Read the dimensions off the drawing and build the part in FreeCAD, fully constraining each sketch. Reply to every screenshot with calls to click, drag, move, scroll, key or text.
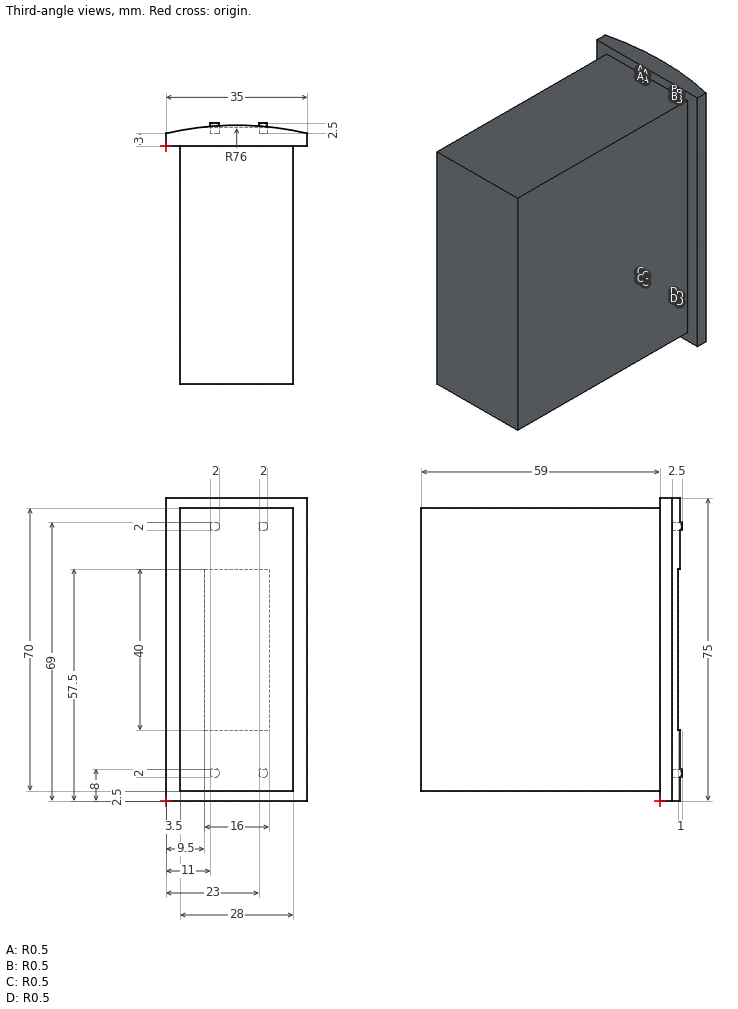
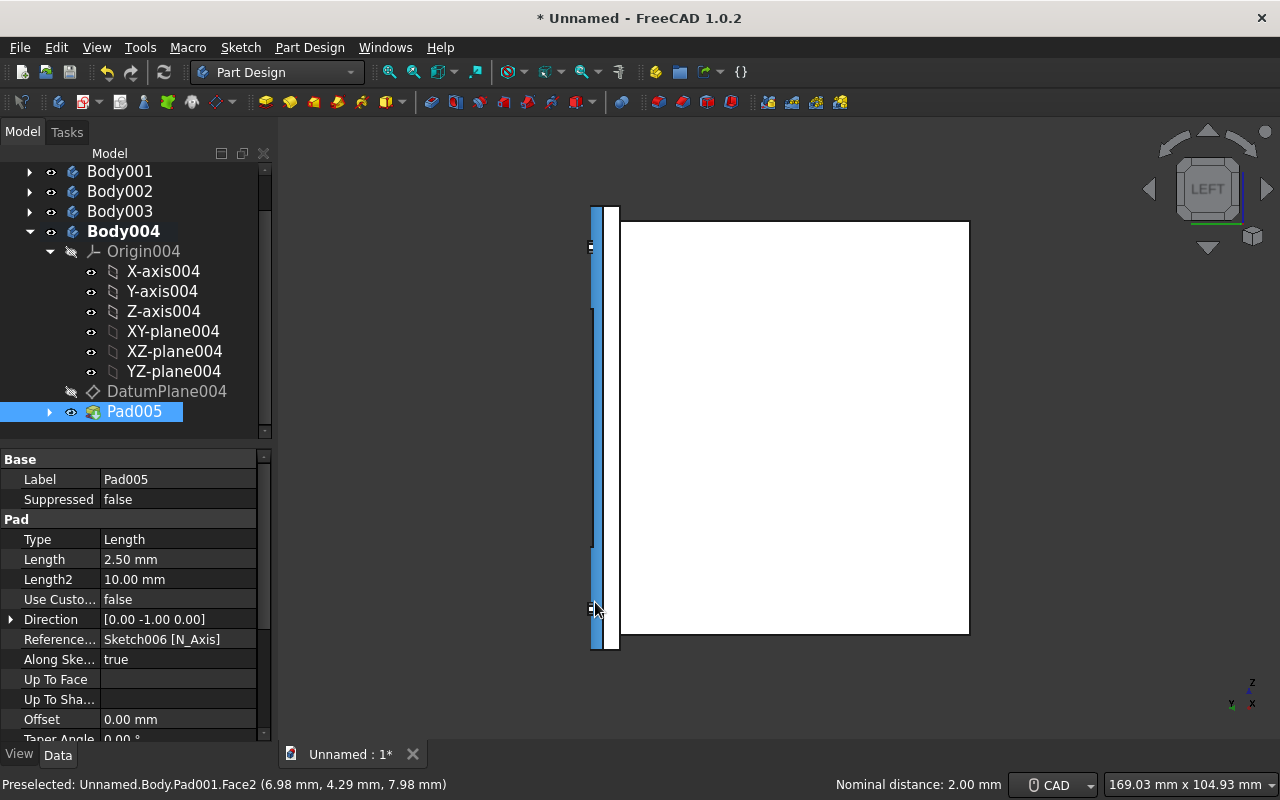
key(v)
key(3)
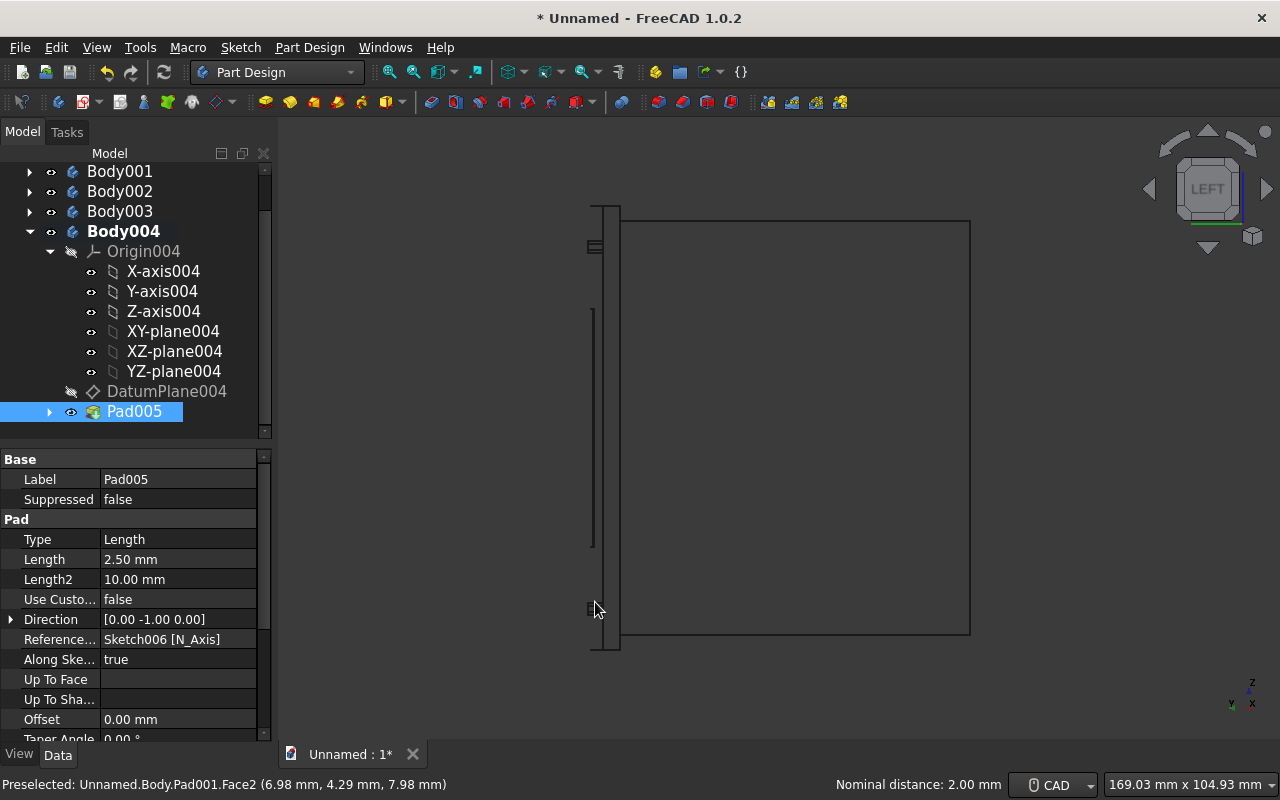
key(0)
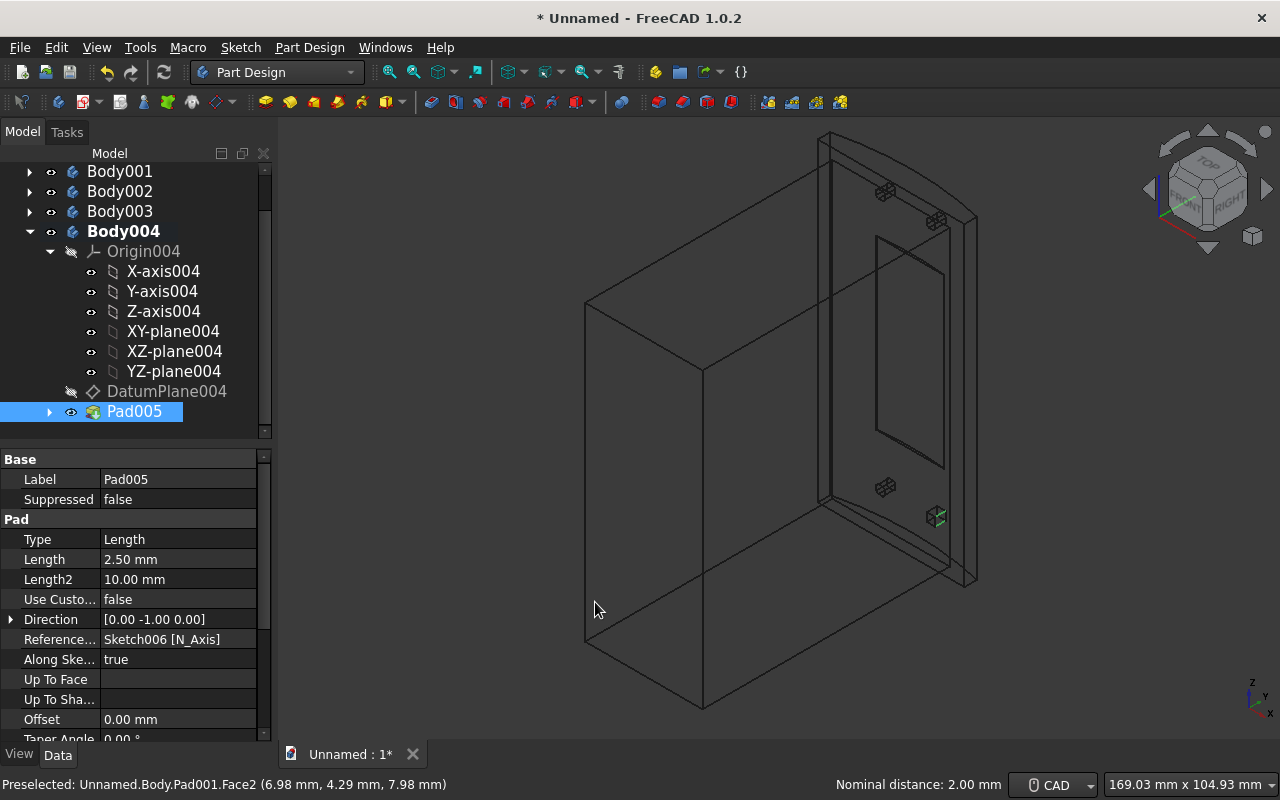
key(v)
key(f)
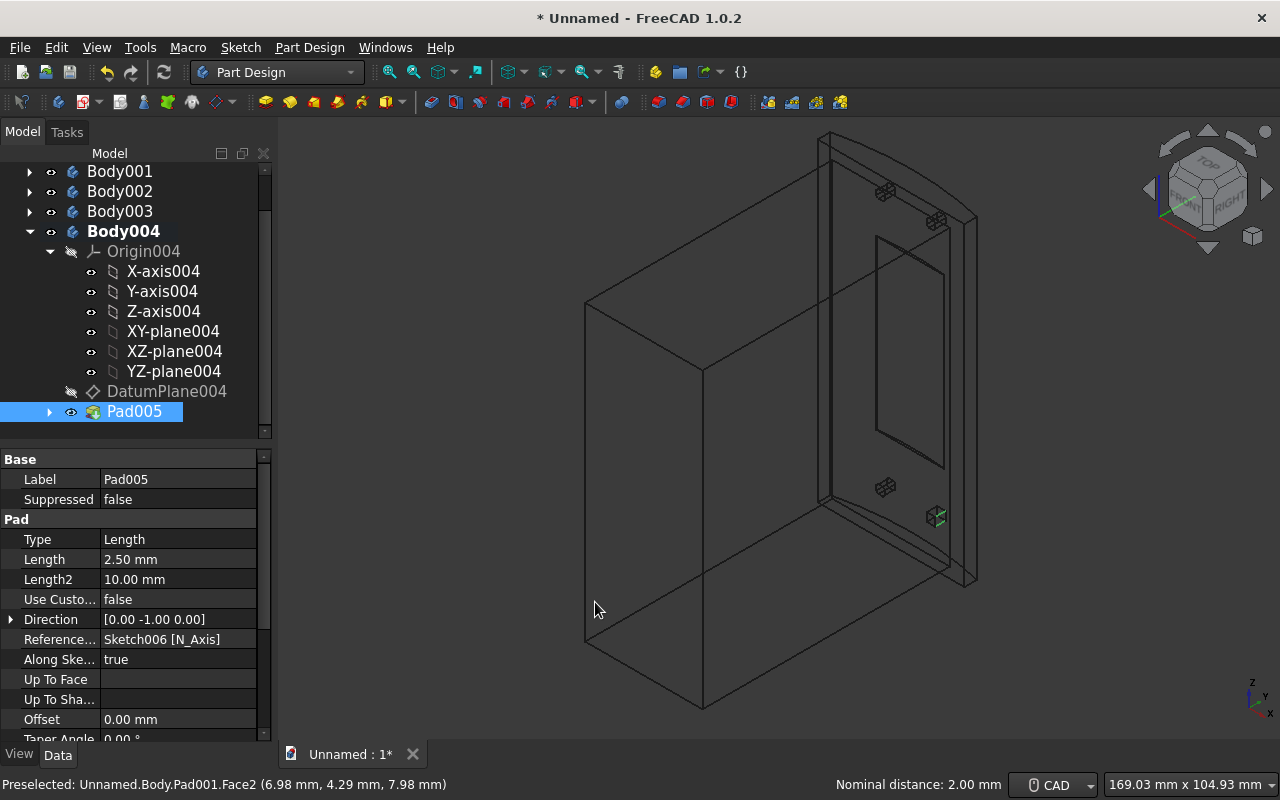
click(933, 507, ctrl)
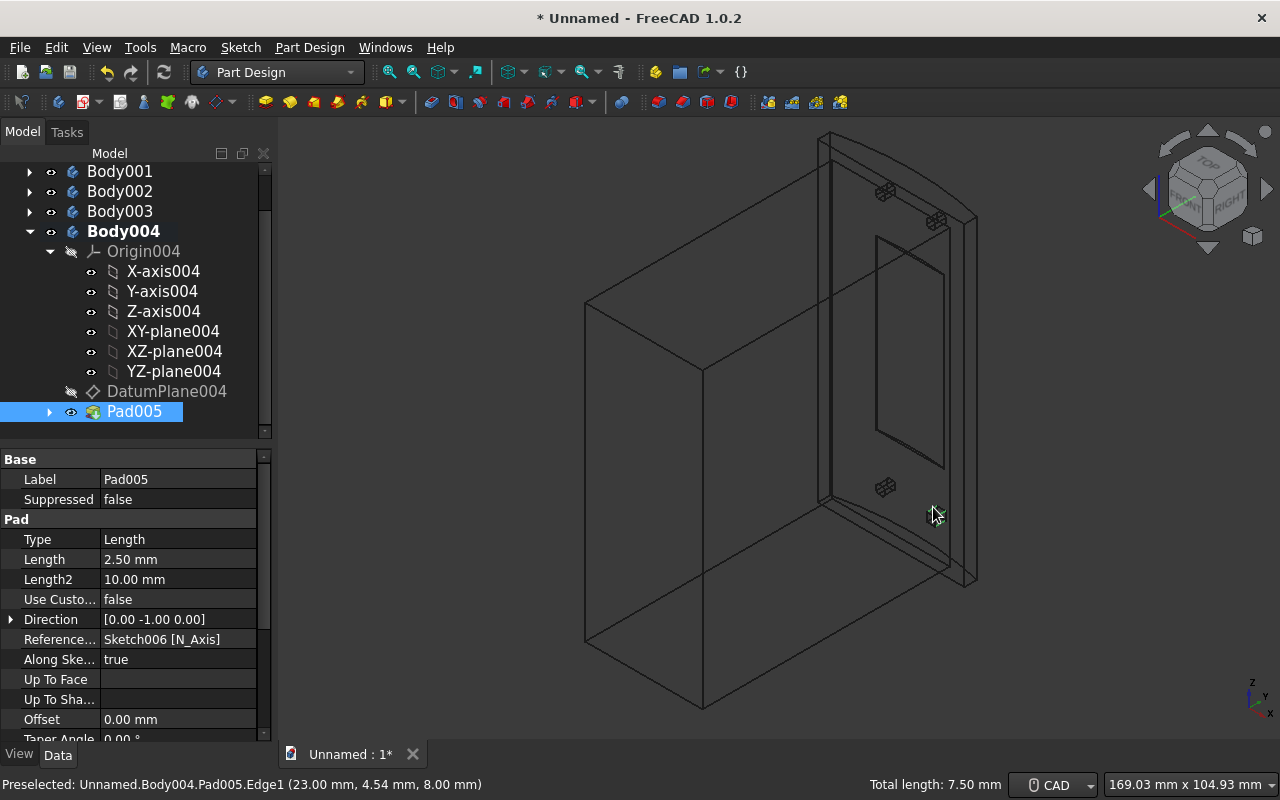
scroll(932, 518, up, 5)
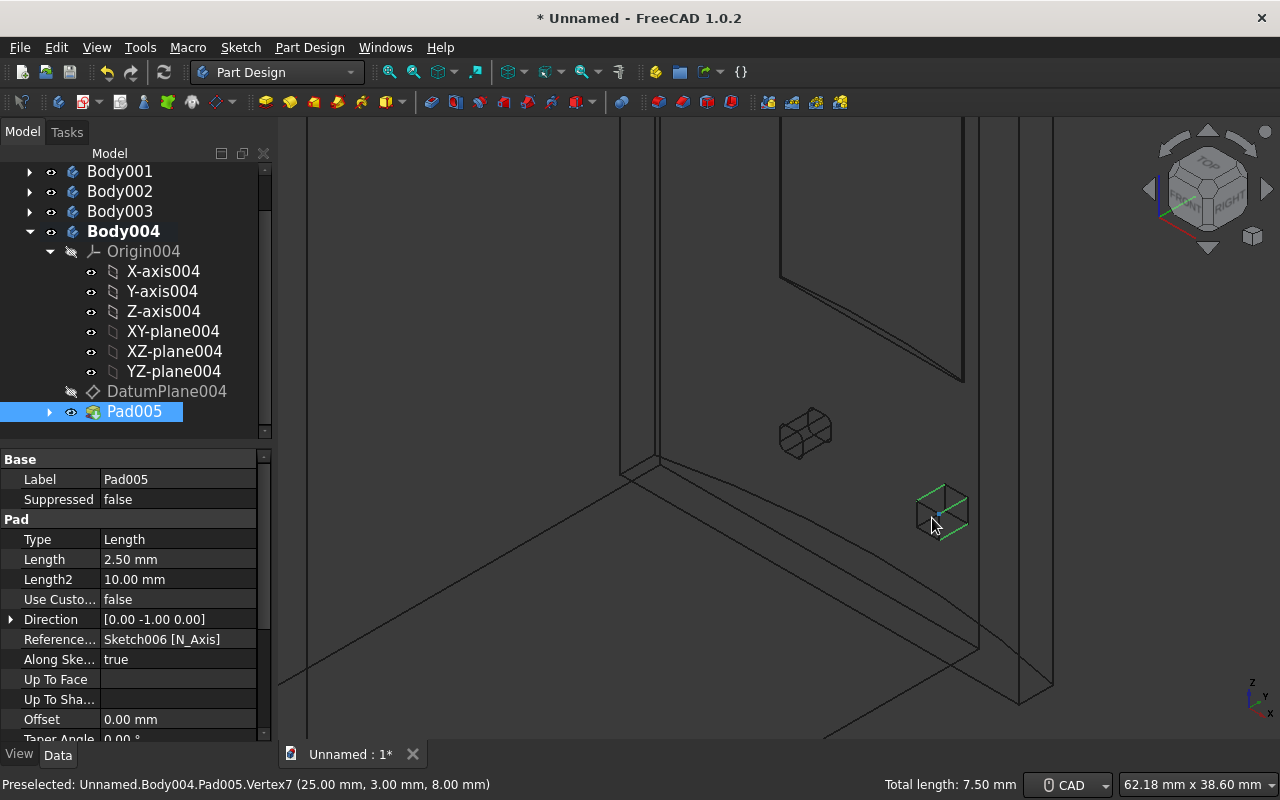
click(931, 518, ctrl)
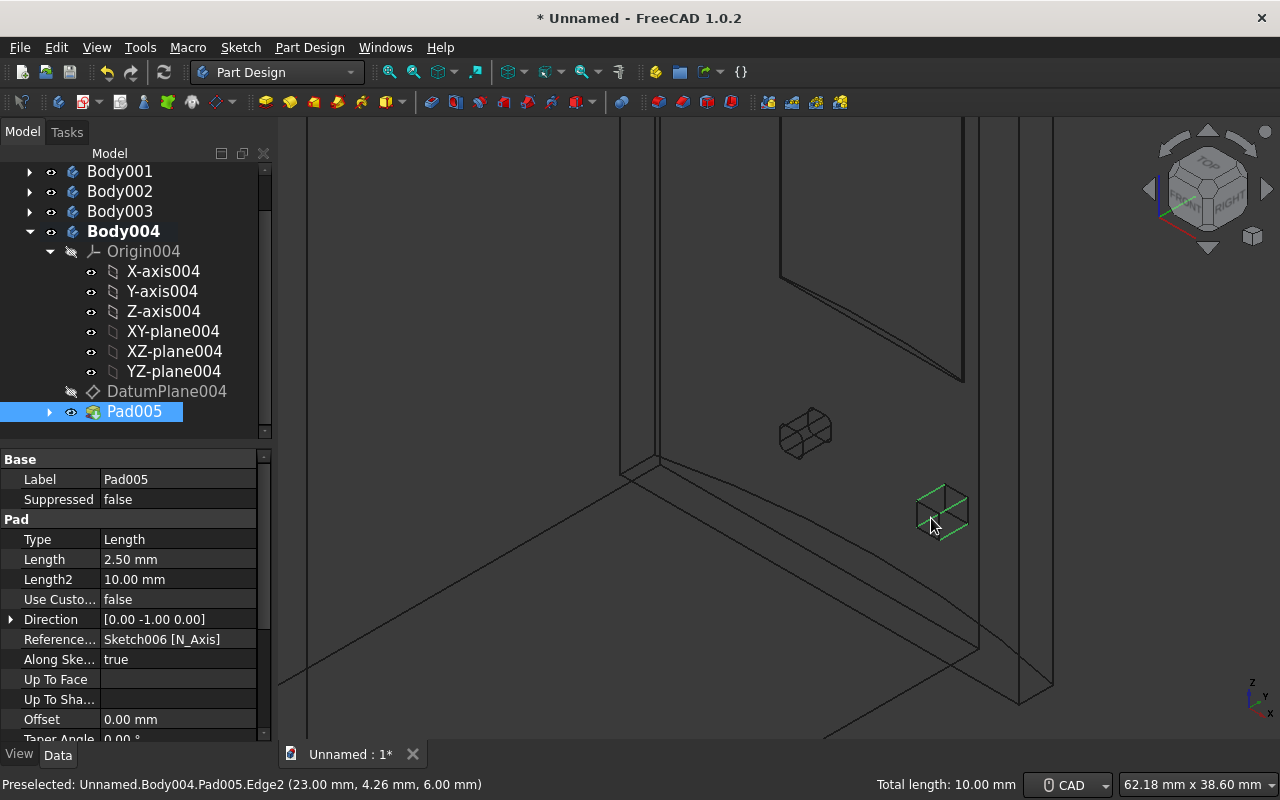
key(v)
key(1)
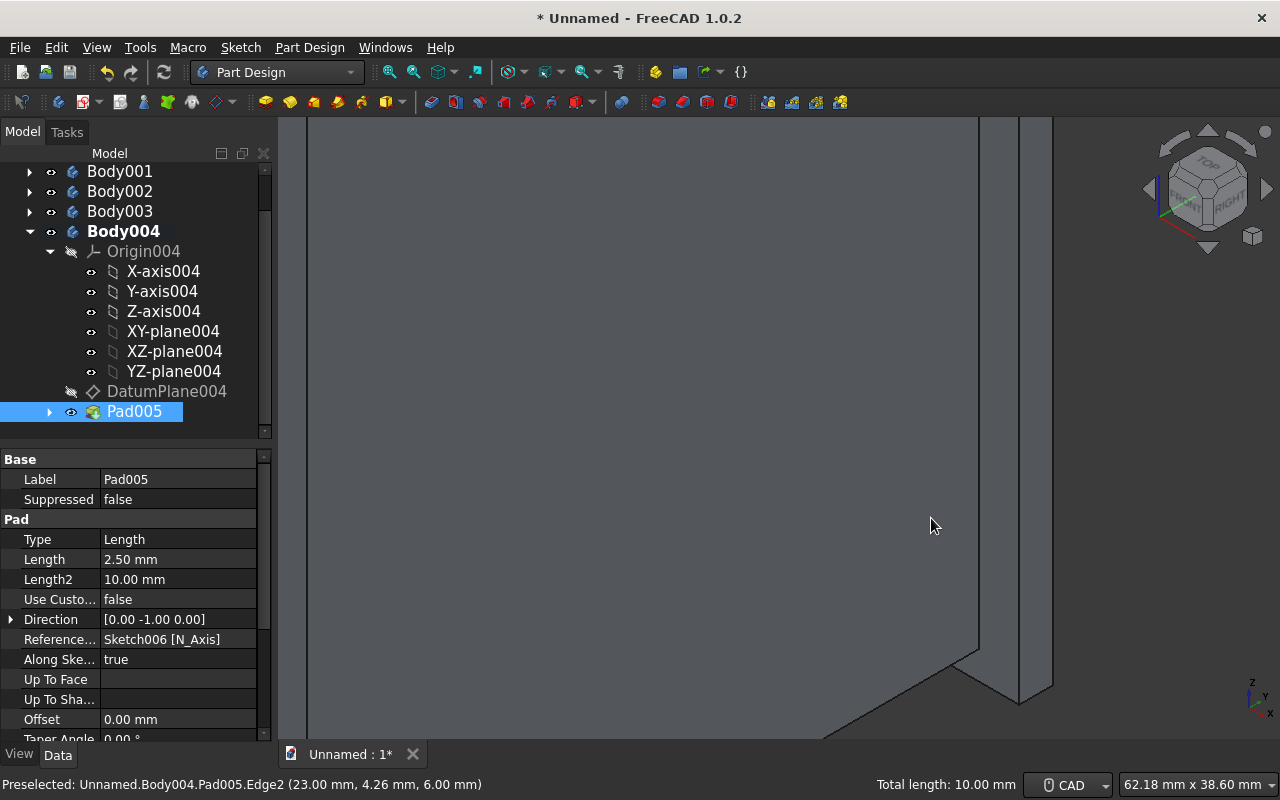
click(660, 102)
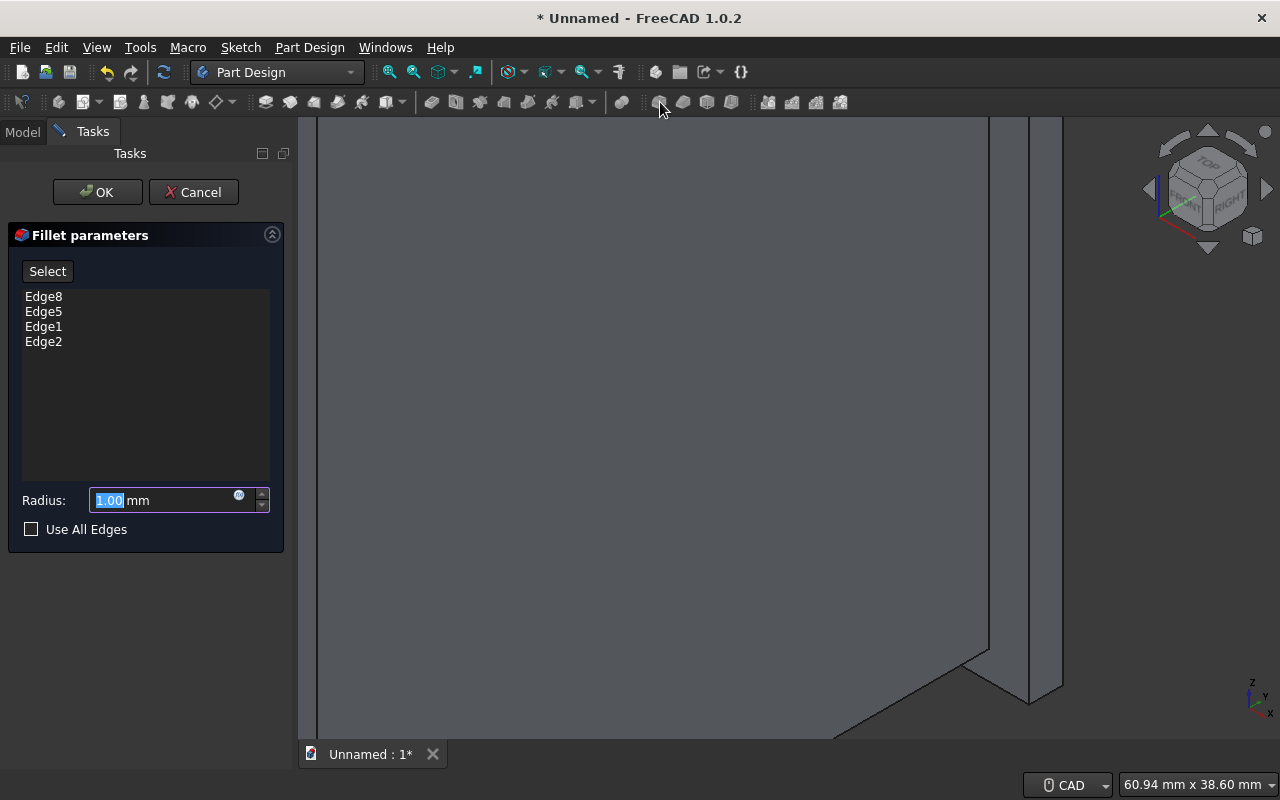
text(0.5)
key(Tab)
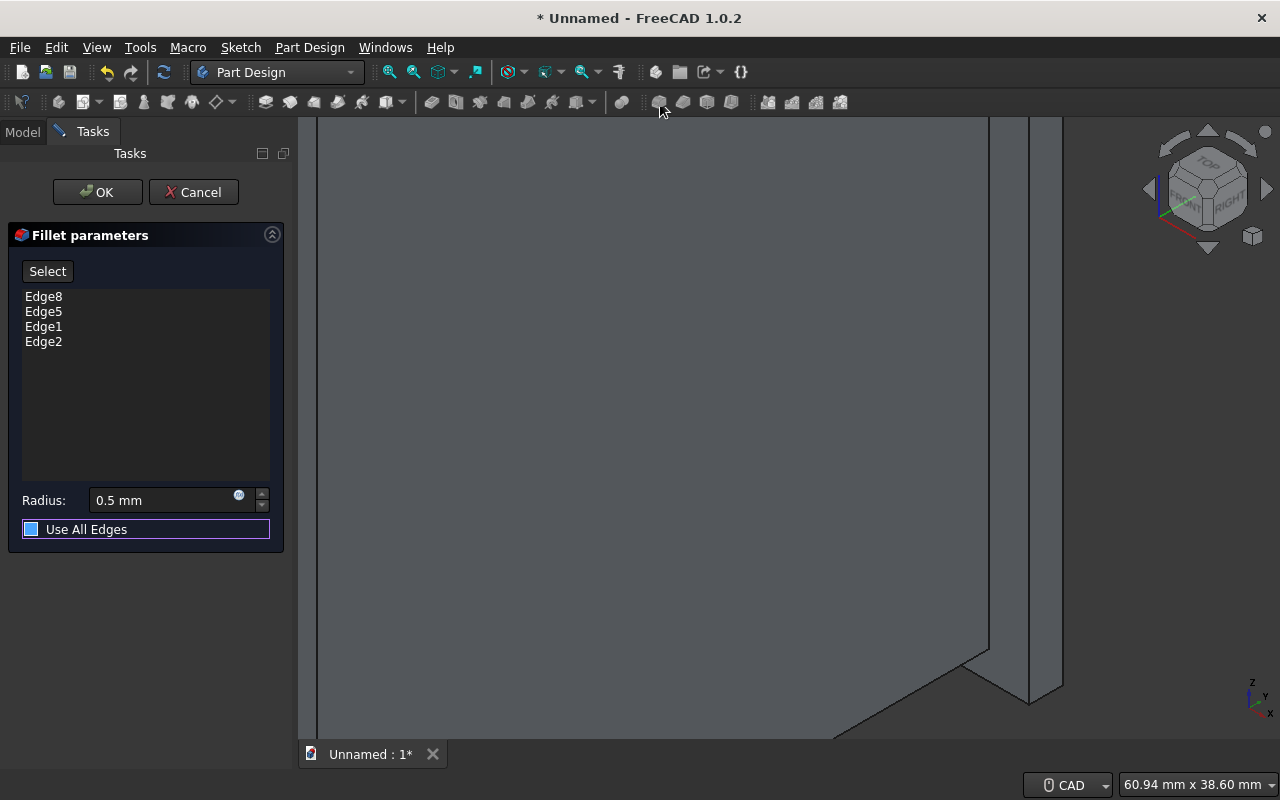
click(98, 192)